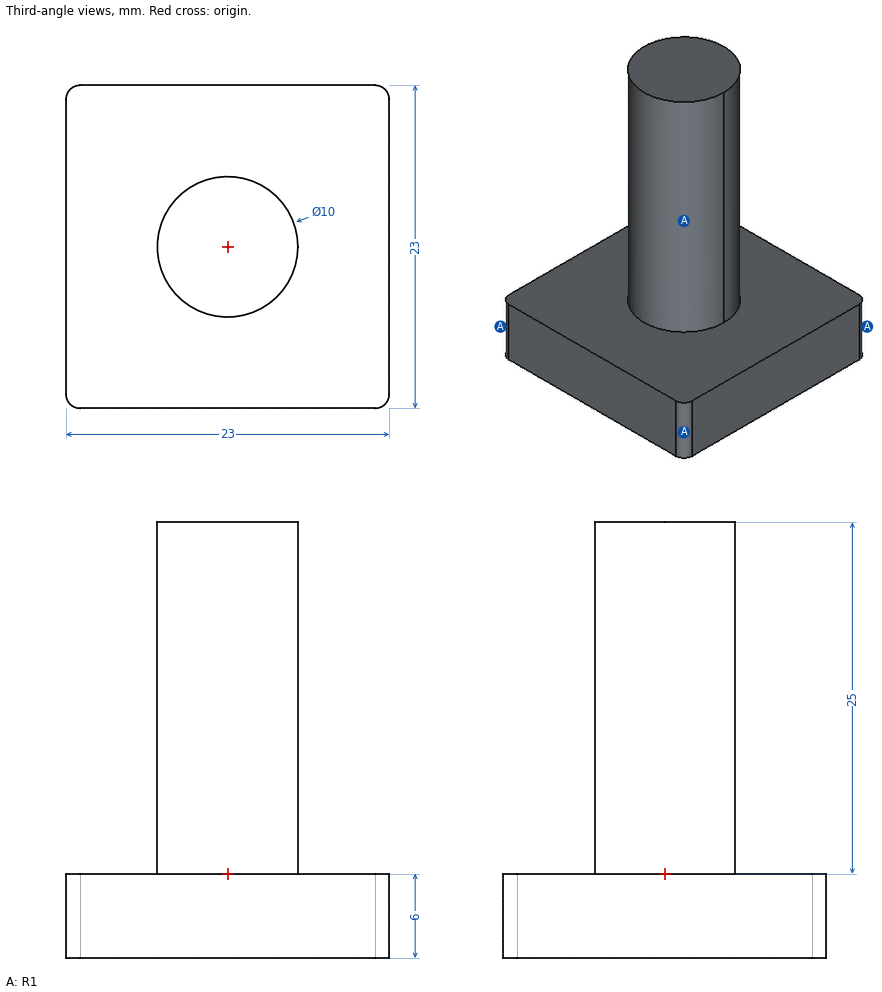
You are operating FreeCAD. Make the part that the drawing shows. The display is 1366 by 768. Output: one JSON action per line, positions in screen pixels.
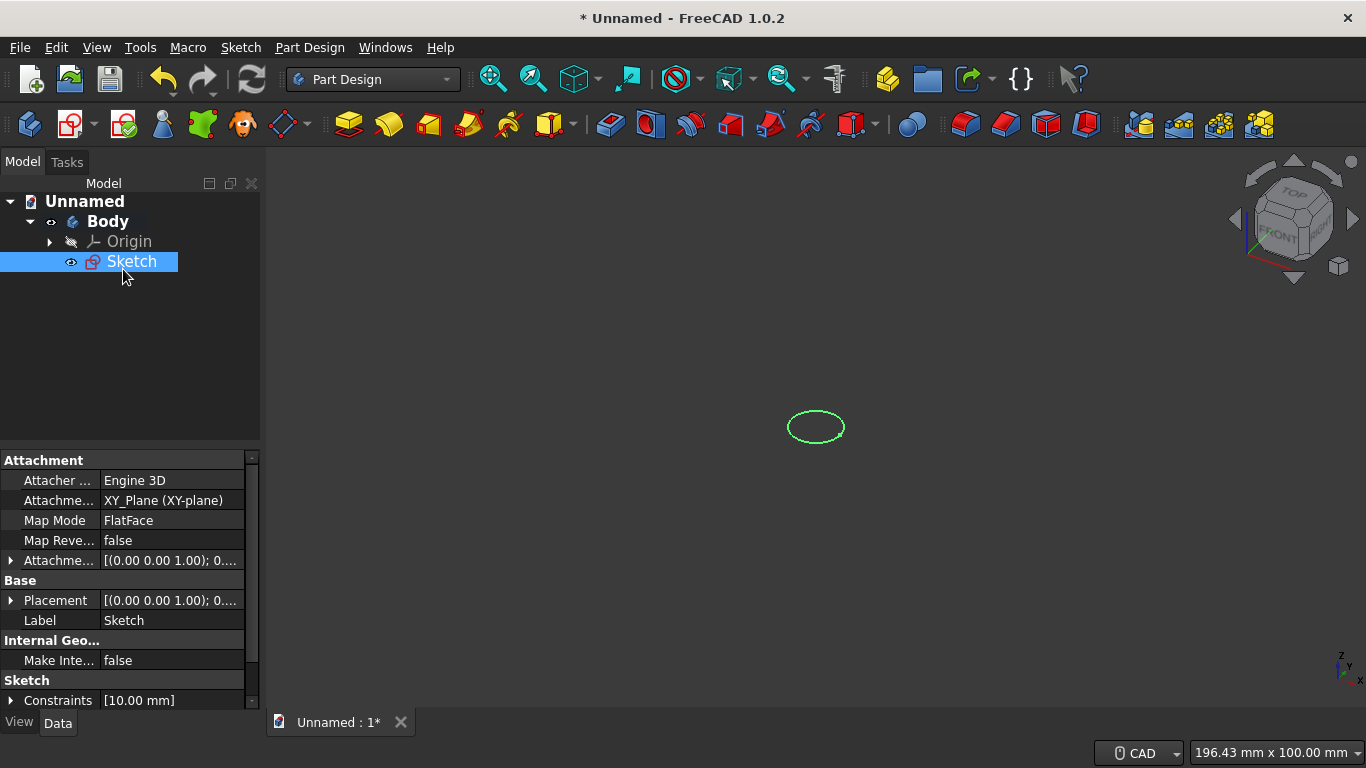
{"action": "left_click", "coordinate": [350, 124]}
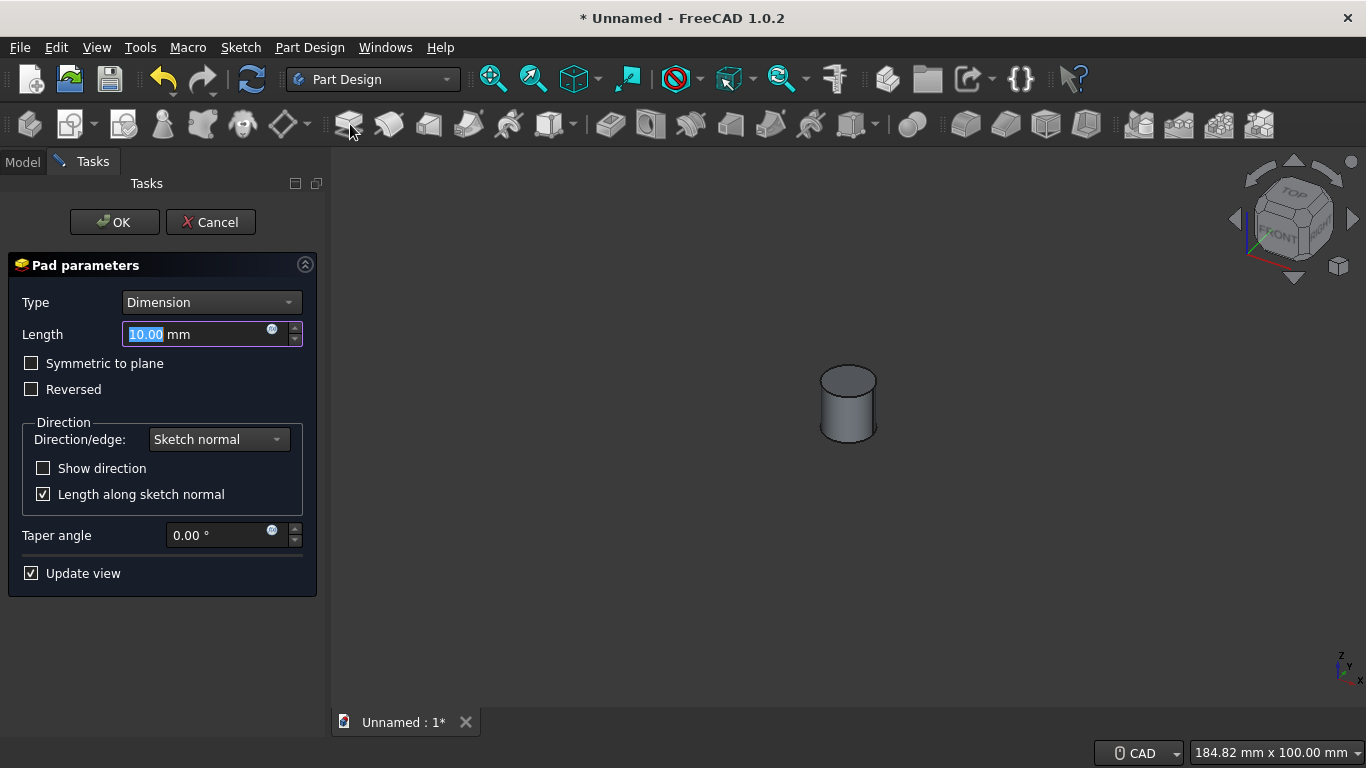
{"action": "type", "text": "25"}
{"action": "key", "text": "Tab"}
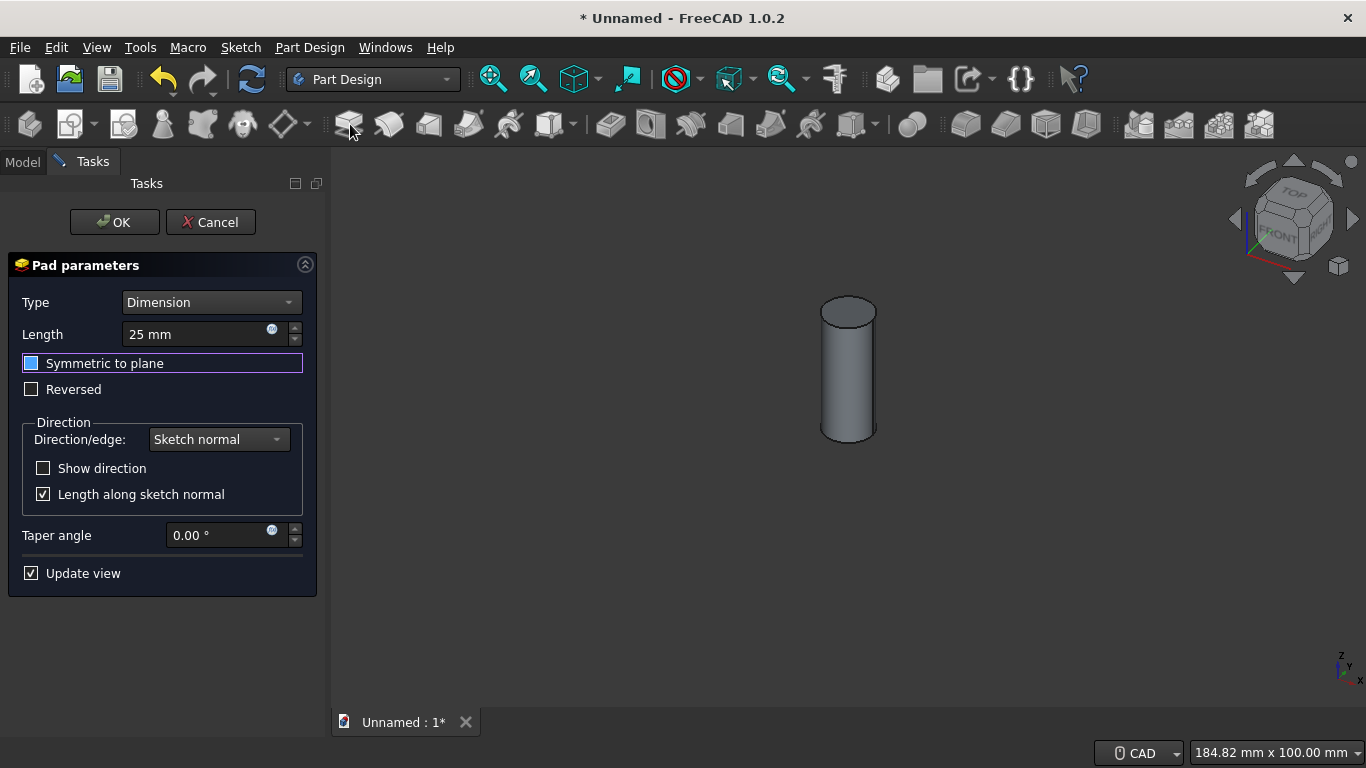
{"action": "left_click", "coordinate": [115, 222]}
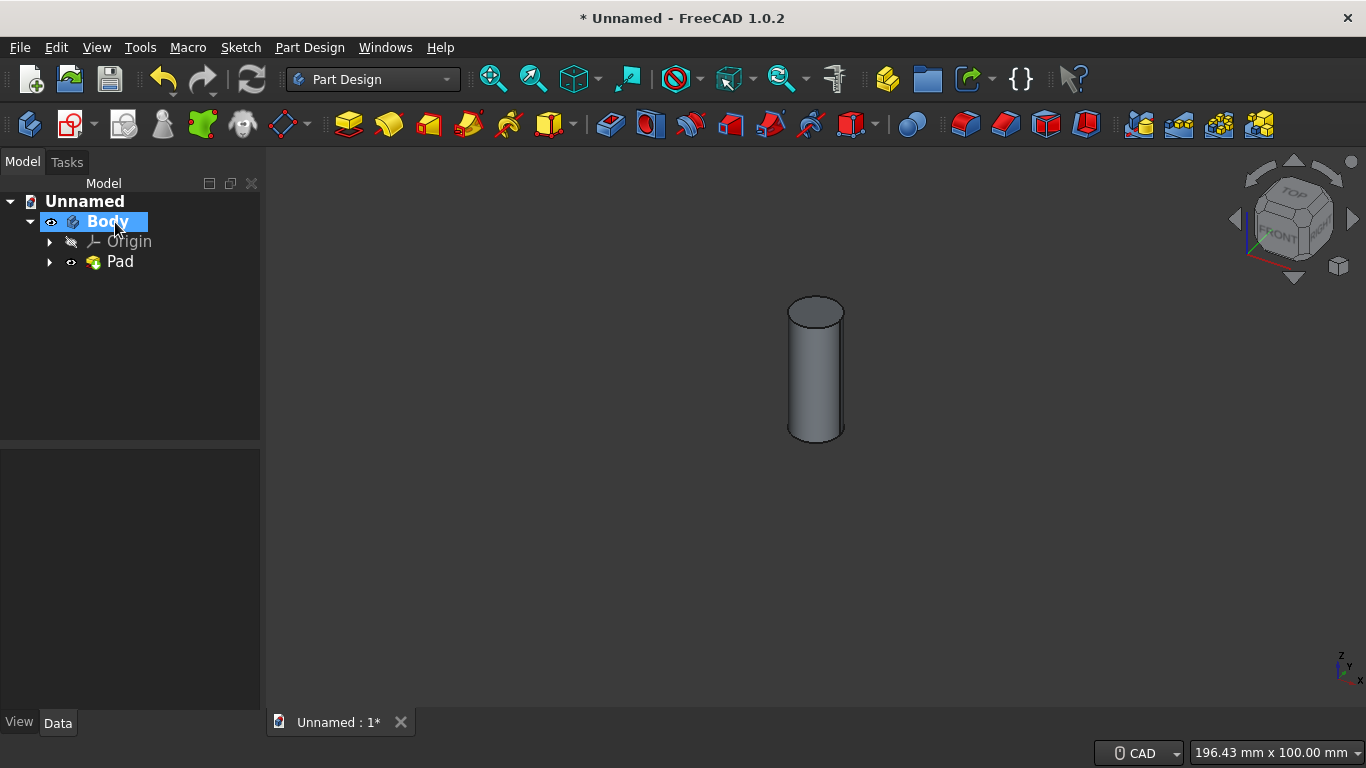
{"action": "left_click", "coordinate": [494, 80]}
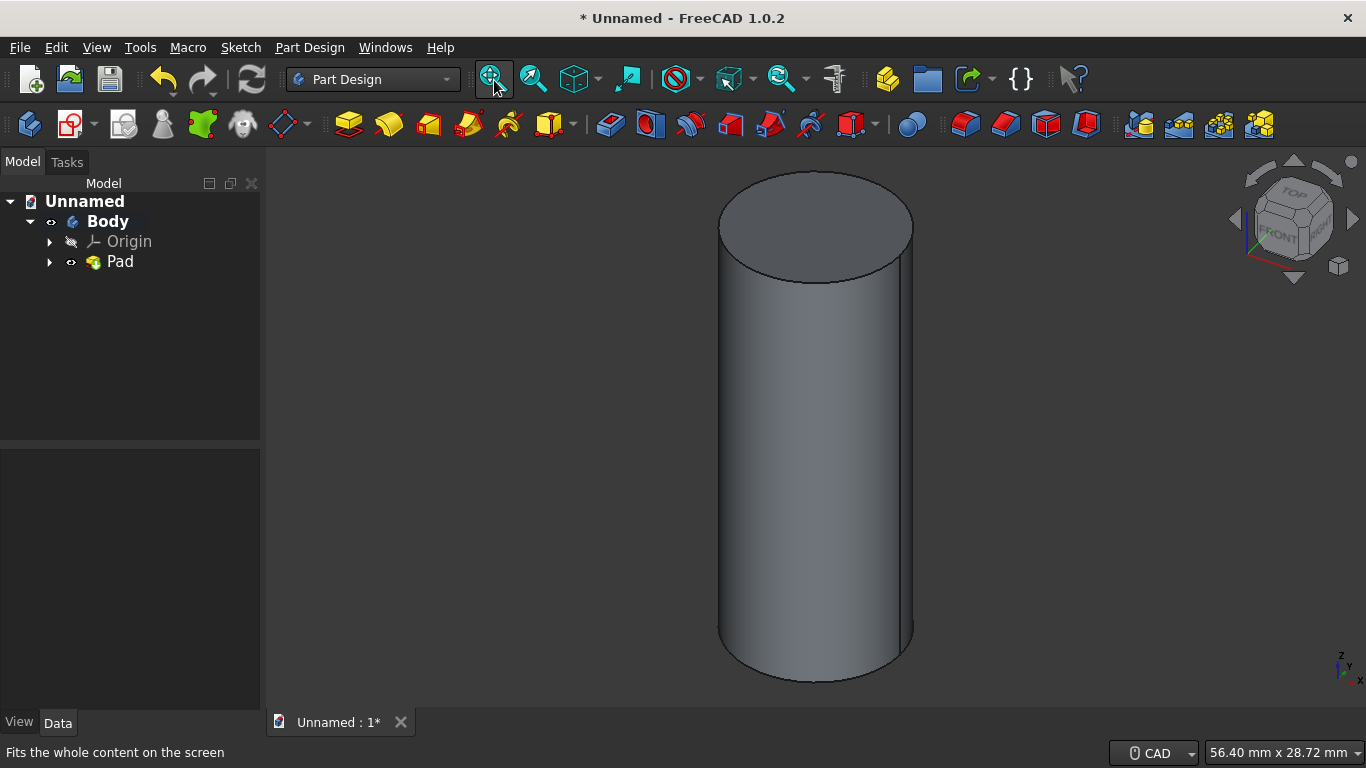
{"action": "left_click", "coordinate": [70, 124]}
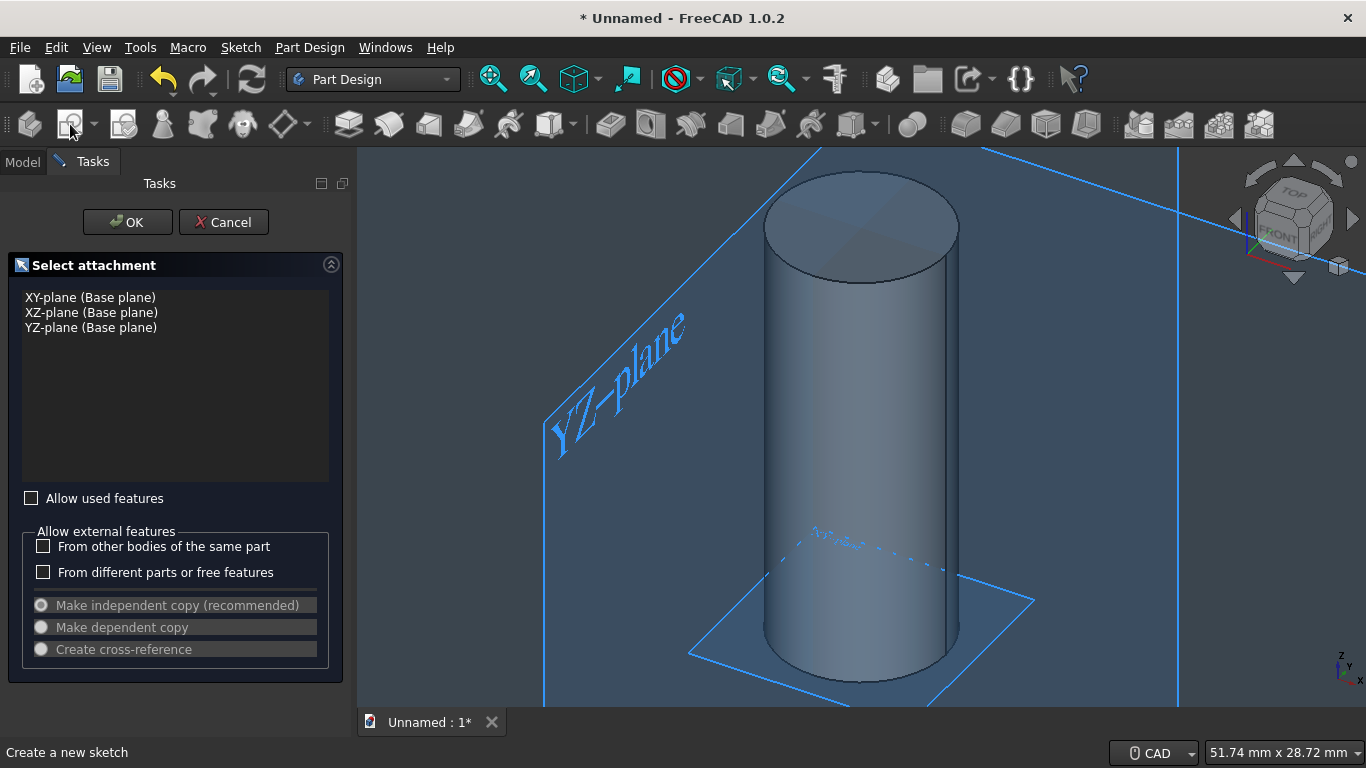
{"action": "left_click", "coordinate": [82, 298]}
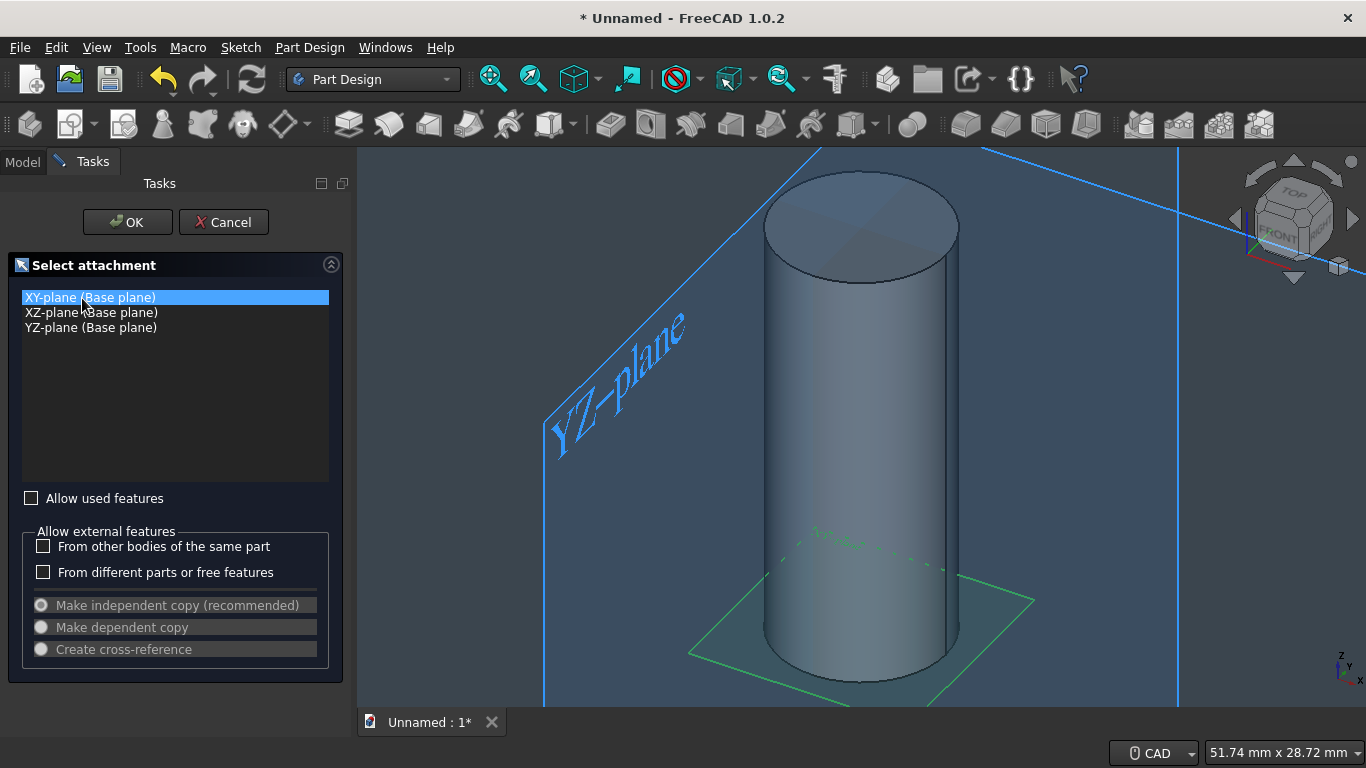
{"action": "left_click", "coordinate": [128, 222]}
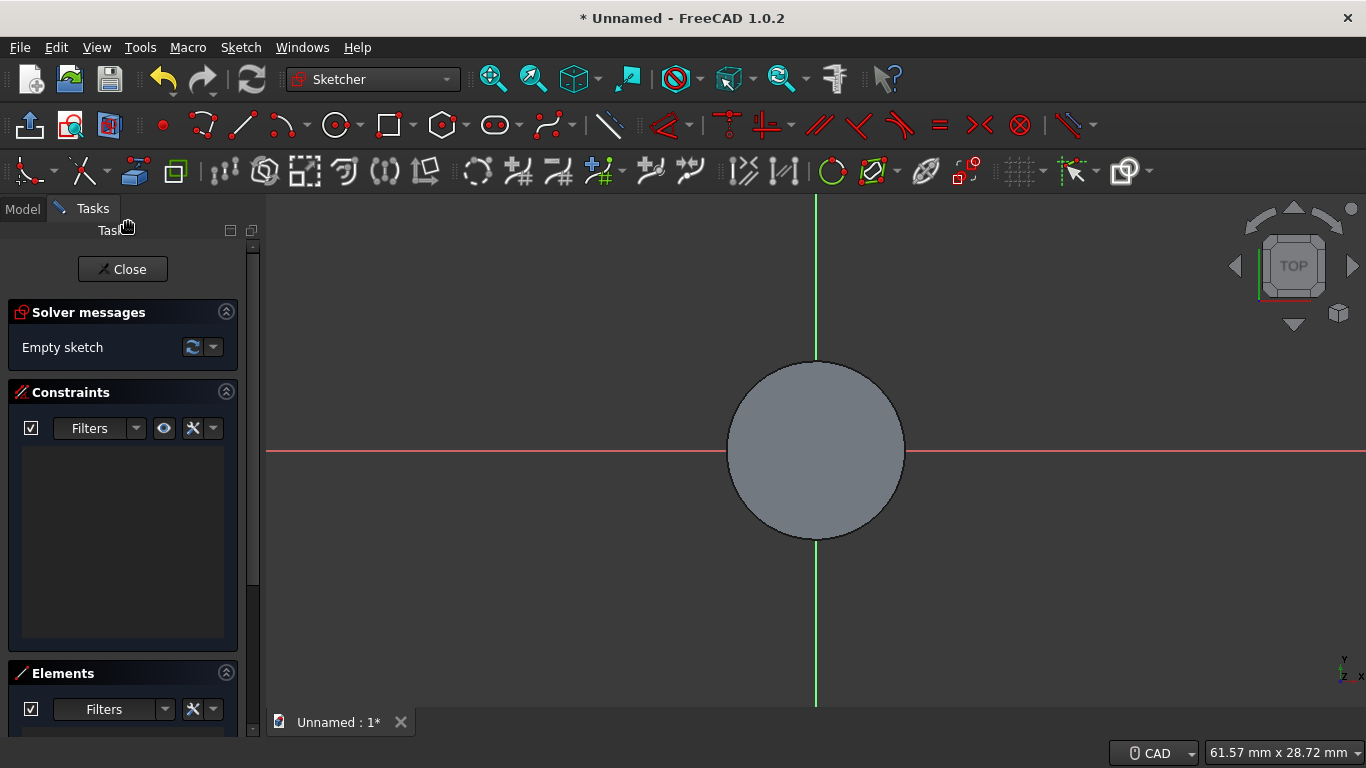
{"action": "left_click", "coordinate": [110, 126]}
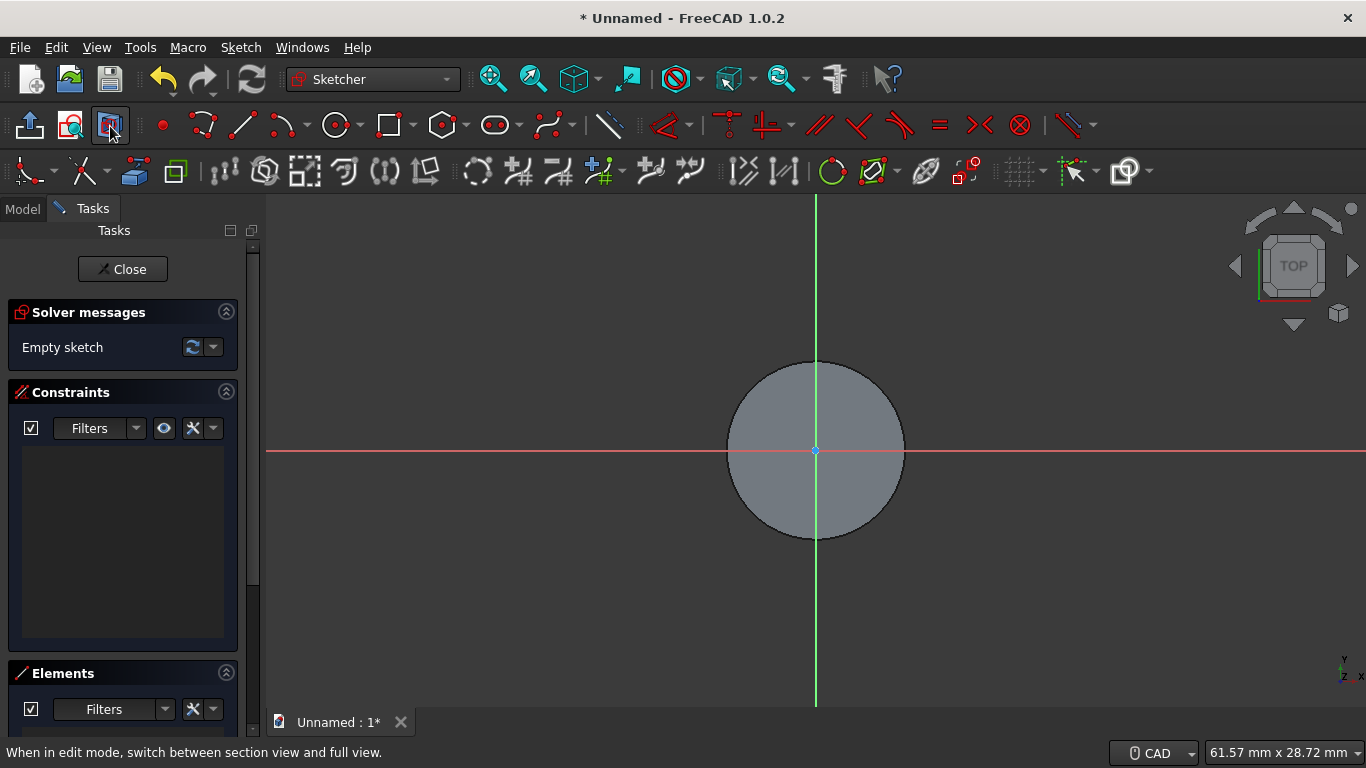
{"action": "scroll", "coordinate": [439, 450], "scroll_direction": "down", "scroll_amount": 1}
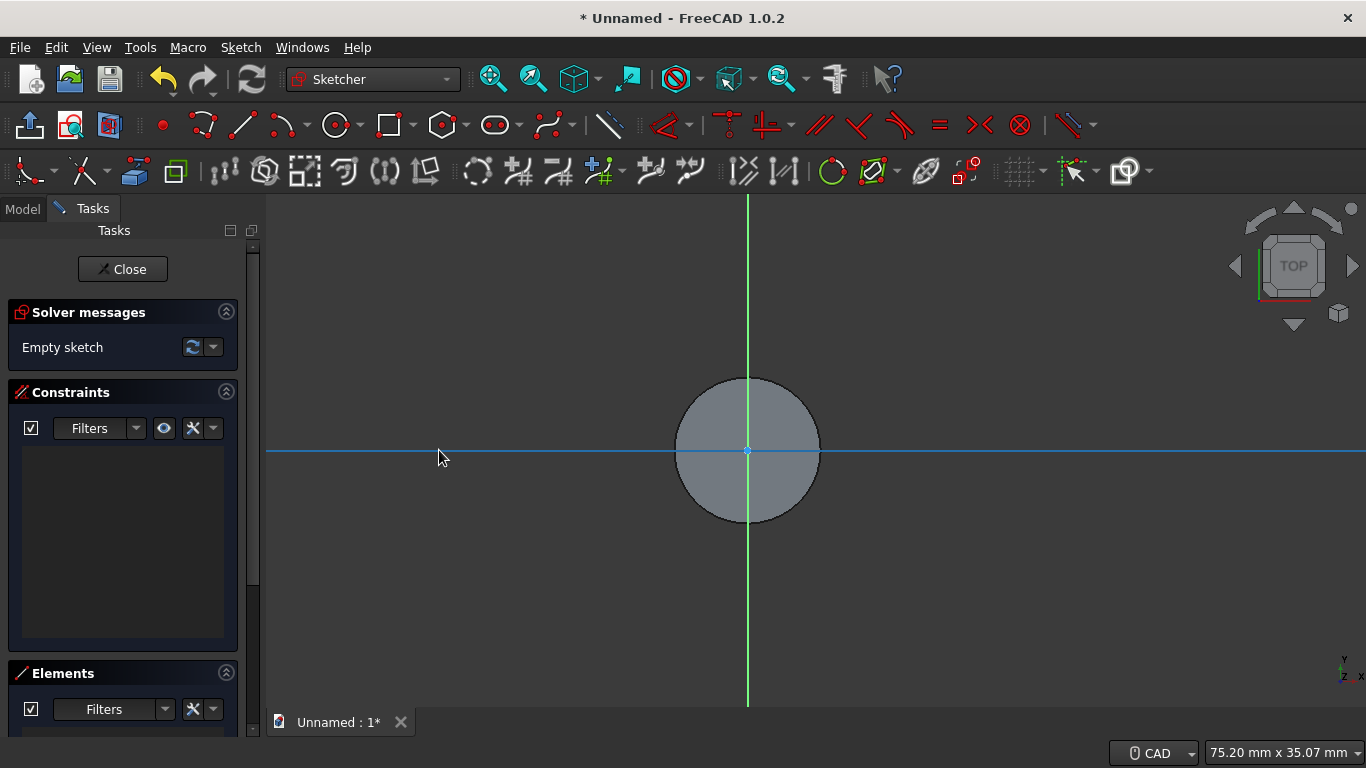
{"action": "key", "text": "g v"}